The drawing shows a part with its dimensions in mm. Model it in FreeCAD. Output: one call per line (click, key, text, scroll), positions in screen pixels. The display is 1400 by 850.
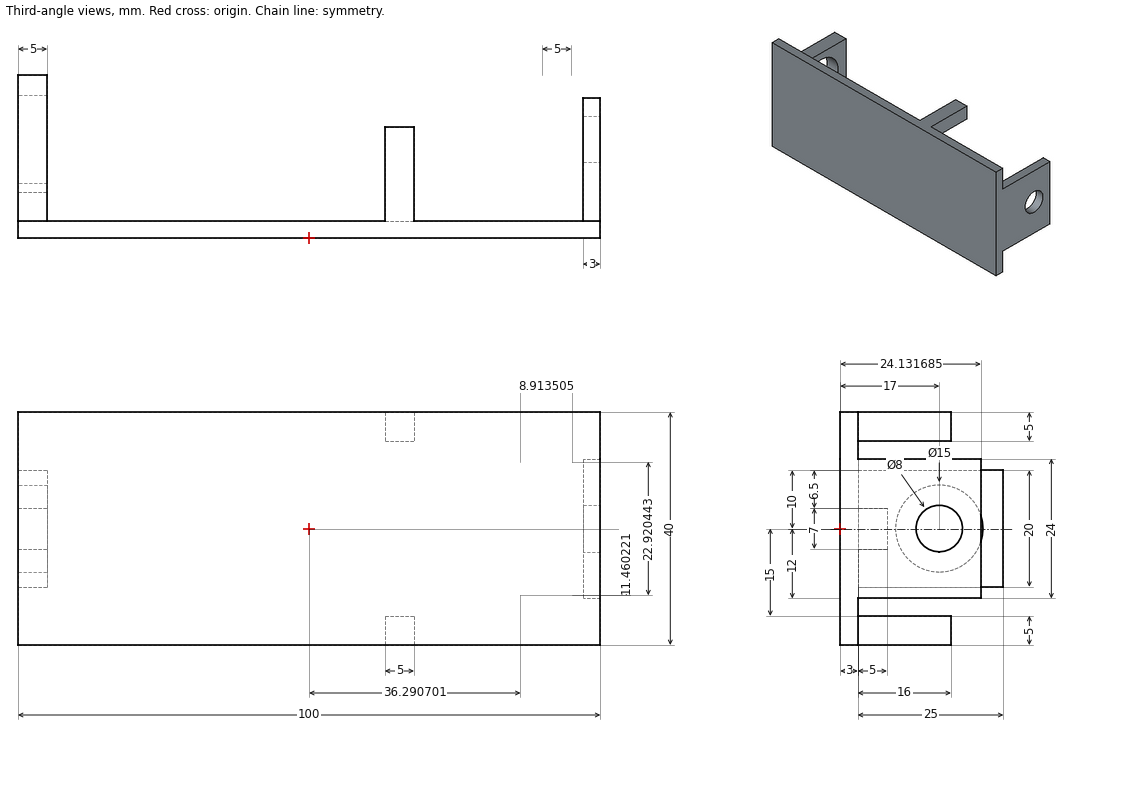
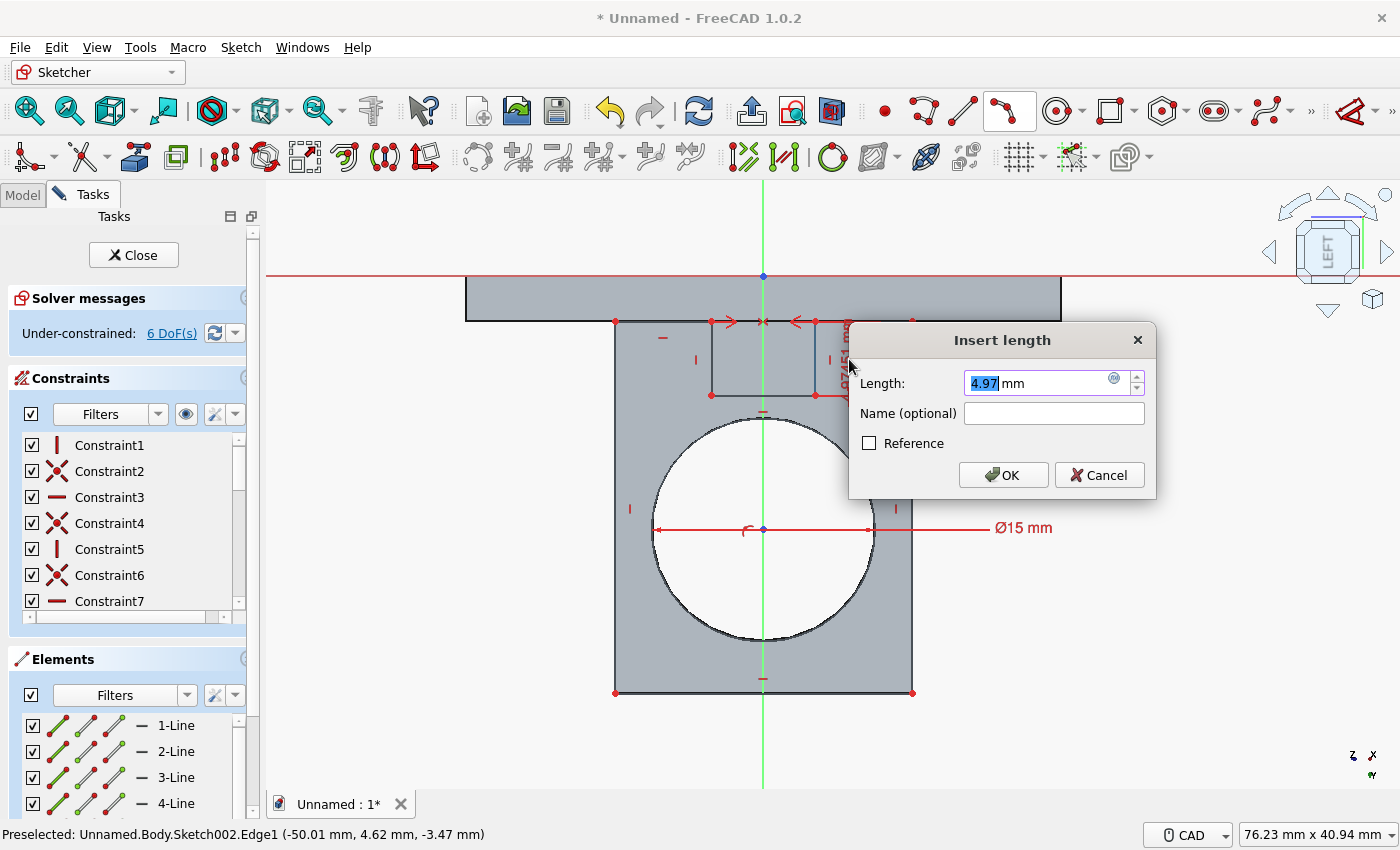
text(5)
key(Return)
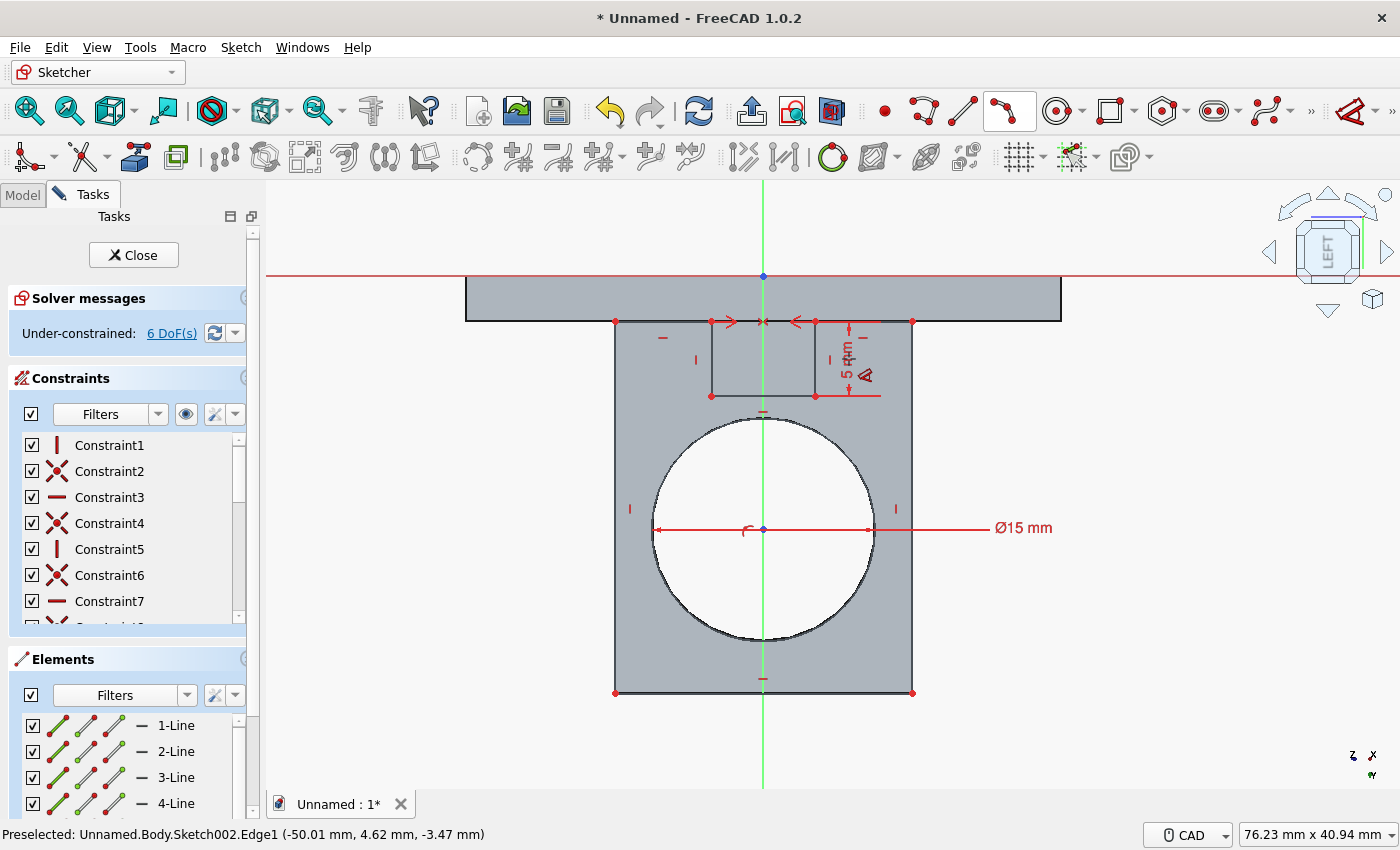
click(784, 396)
click(740, 362)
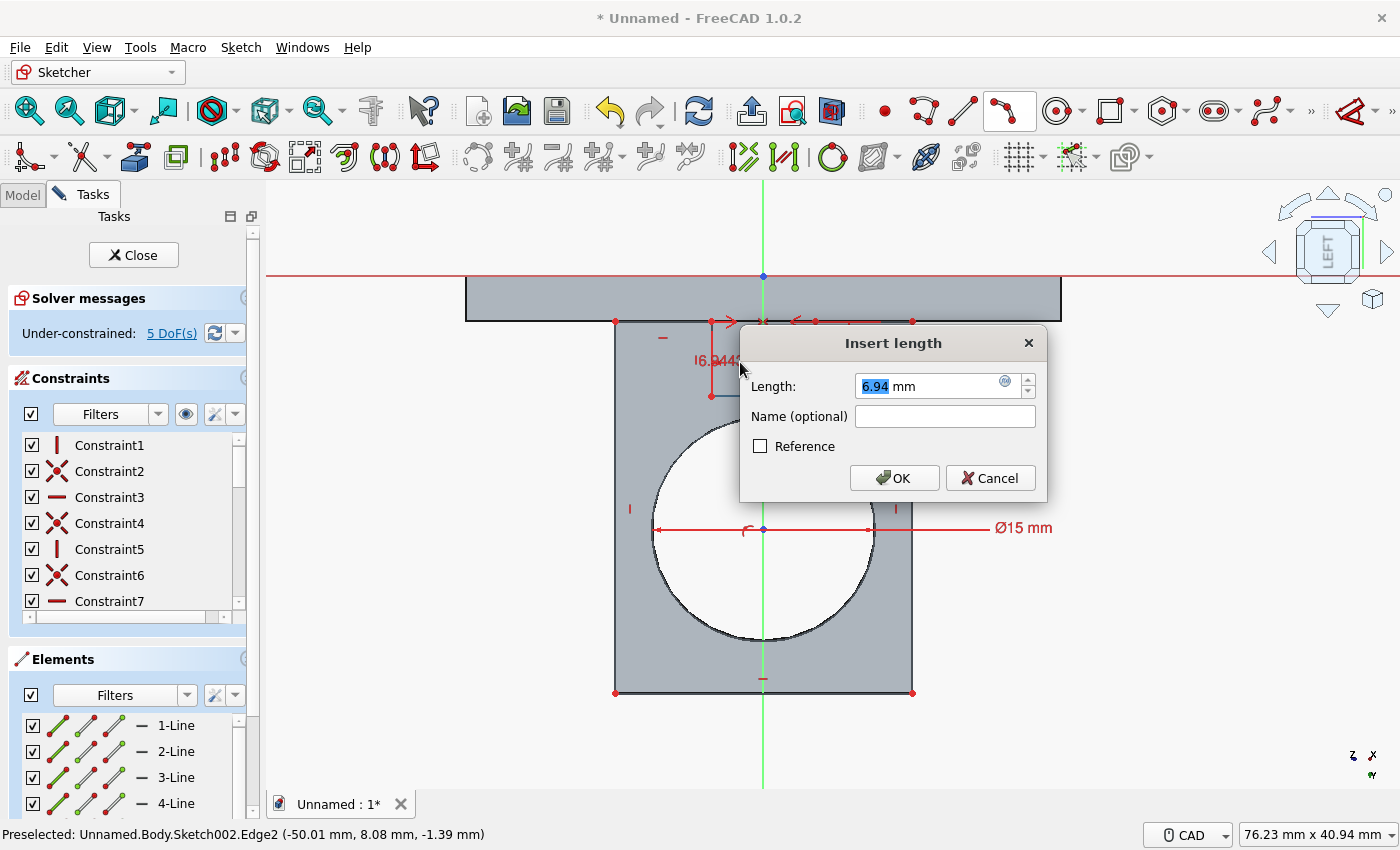
text(7)
key(Return)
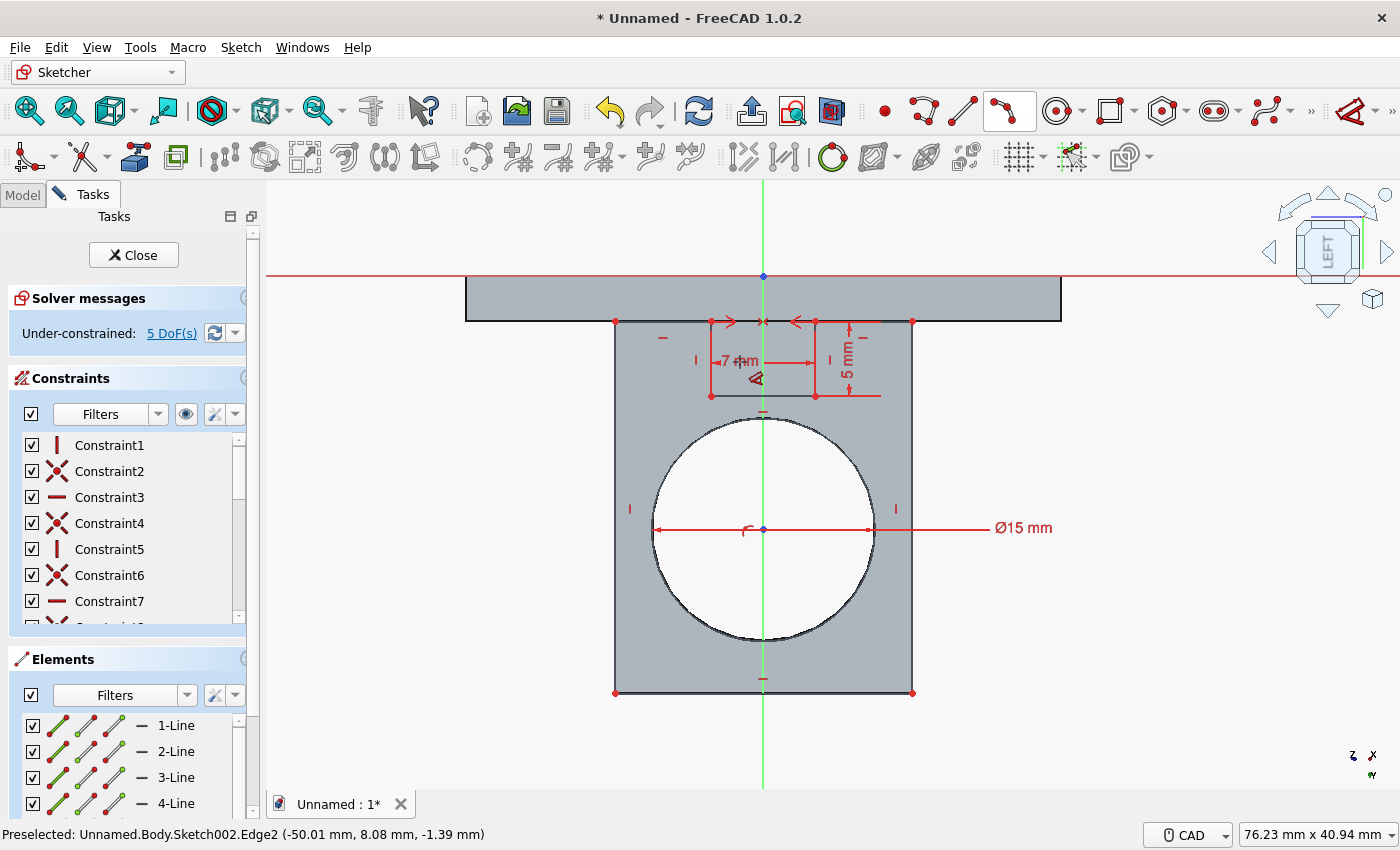
click(615, 434)
click(581, 508)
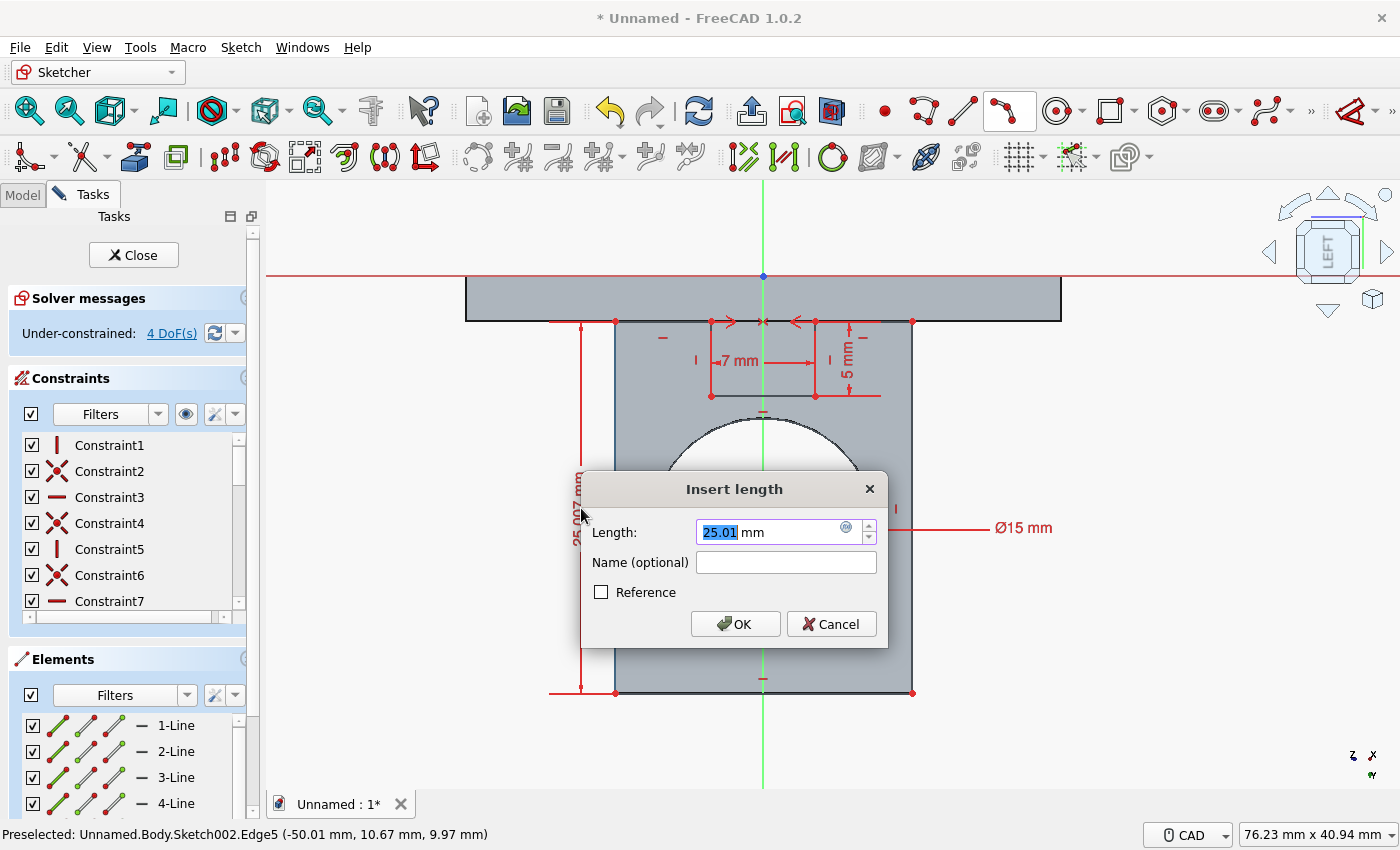
text(25)
key(Return)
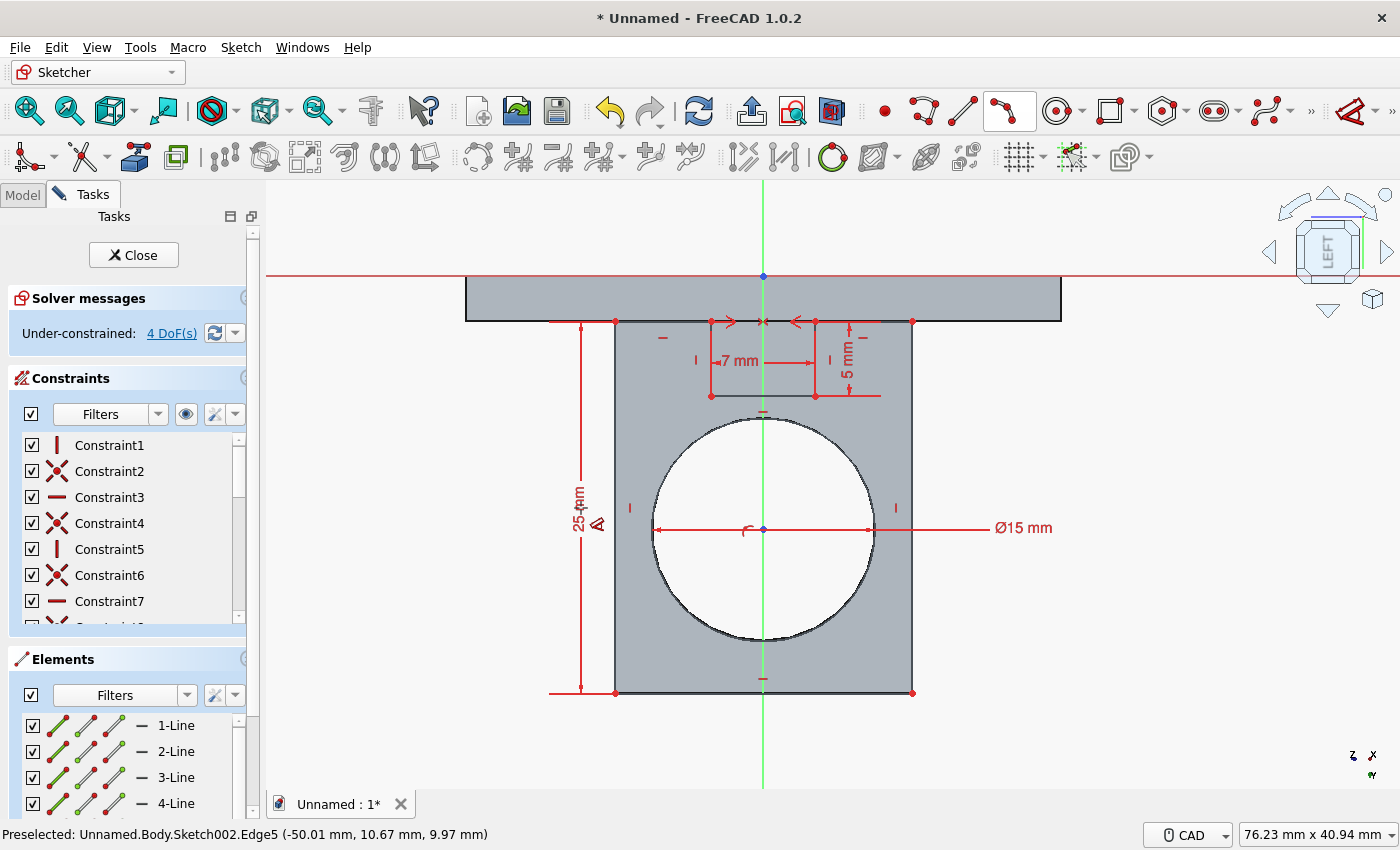
click(704, 694)
click(695, 728)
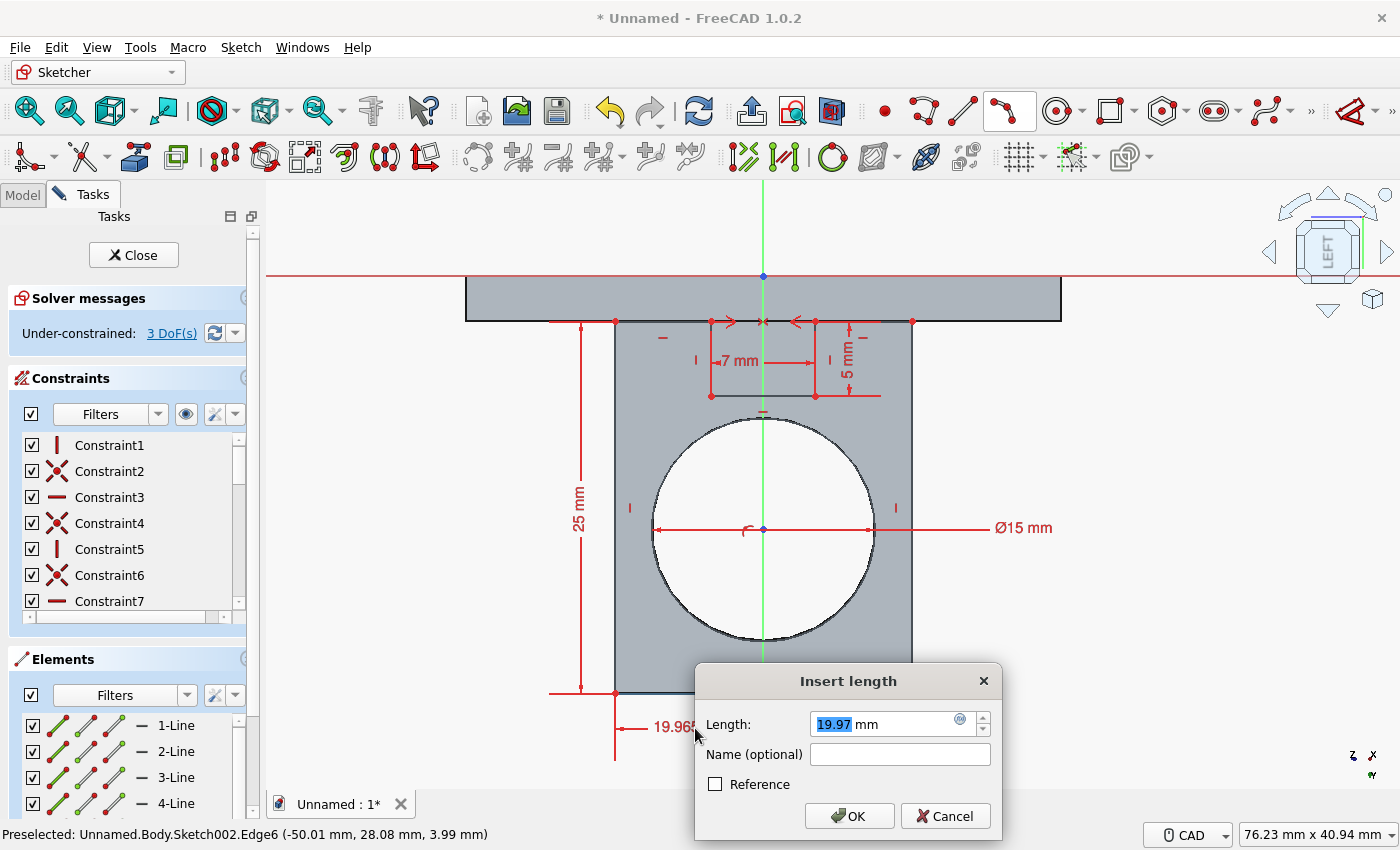
text(20)
key(Return)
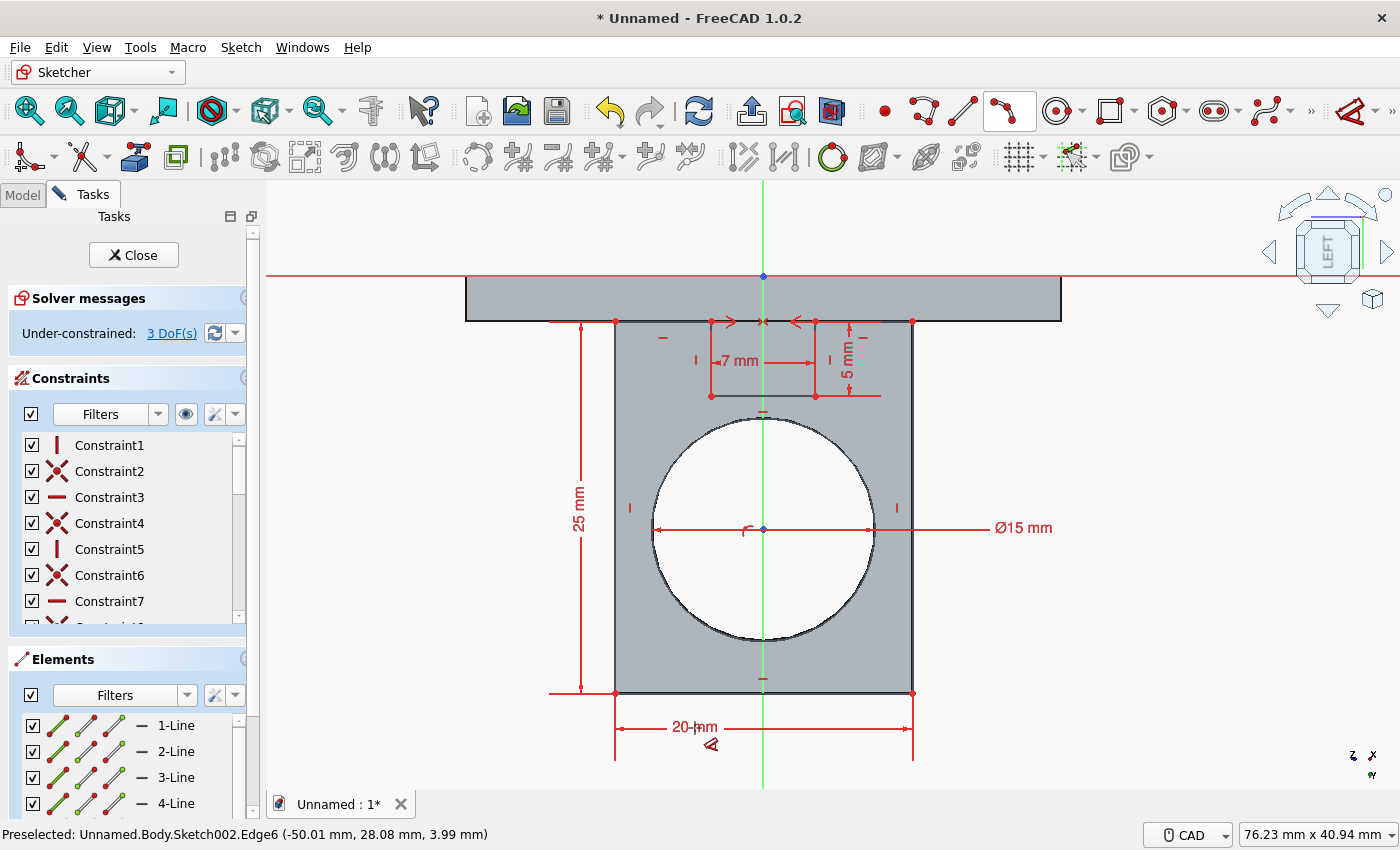
click(815, 322)
click(849, 299)